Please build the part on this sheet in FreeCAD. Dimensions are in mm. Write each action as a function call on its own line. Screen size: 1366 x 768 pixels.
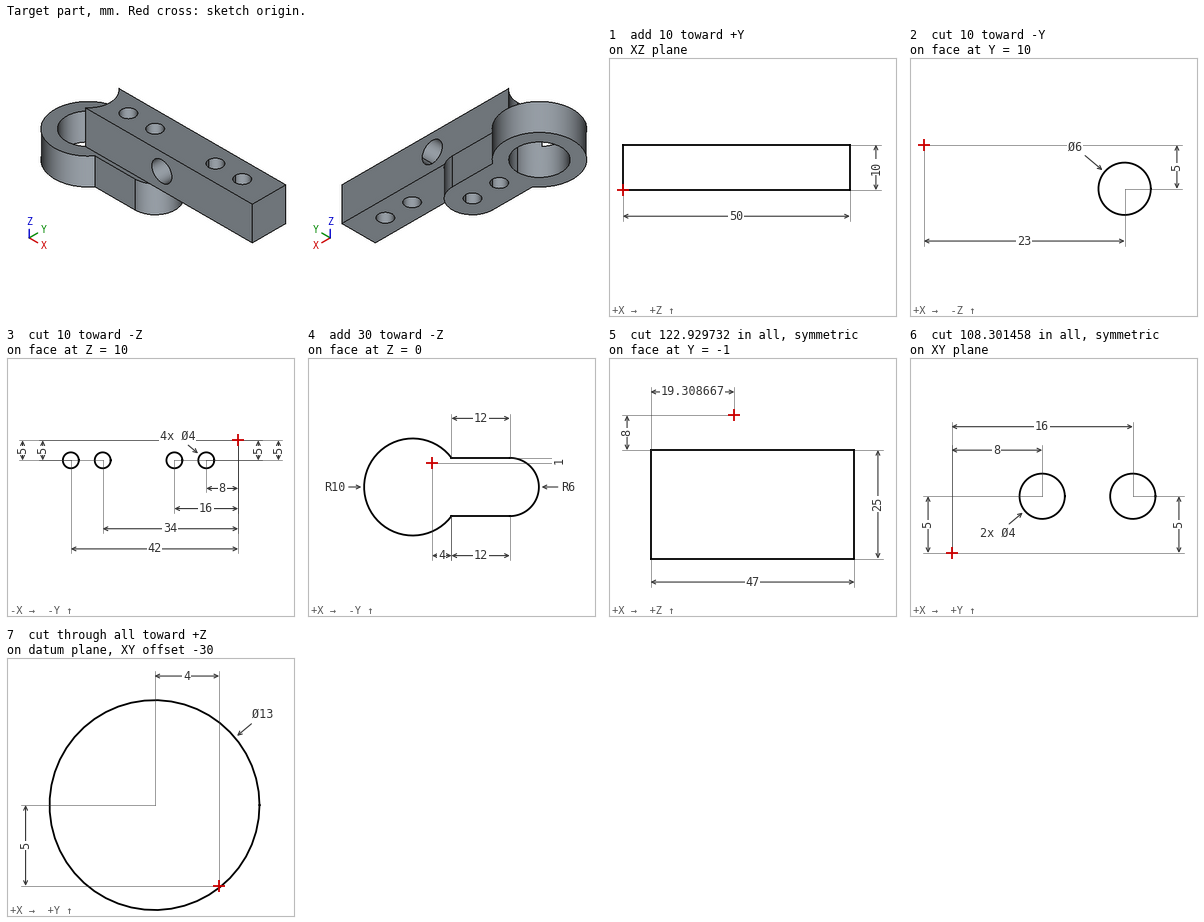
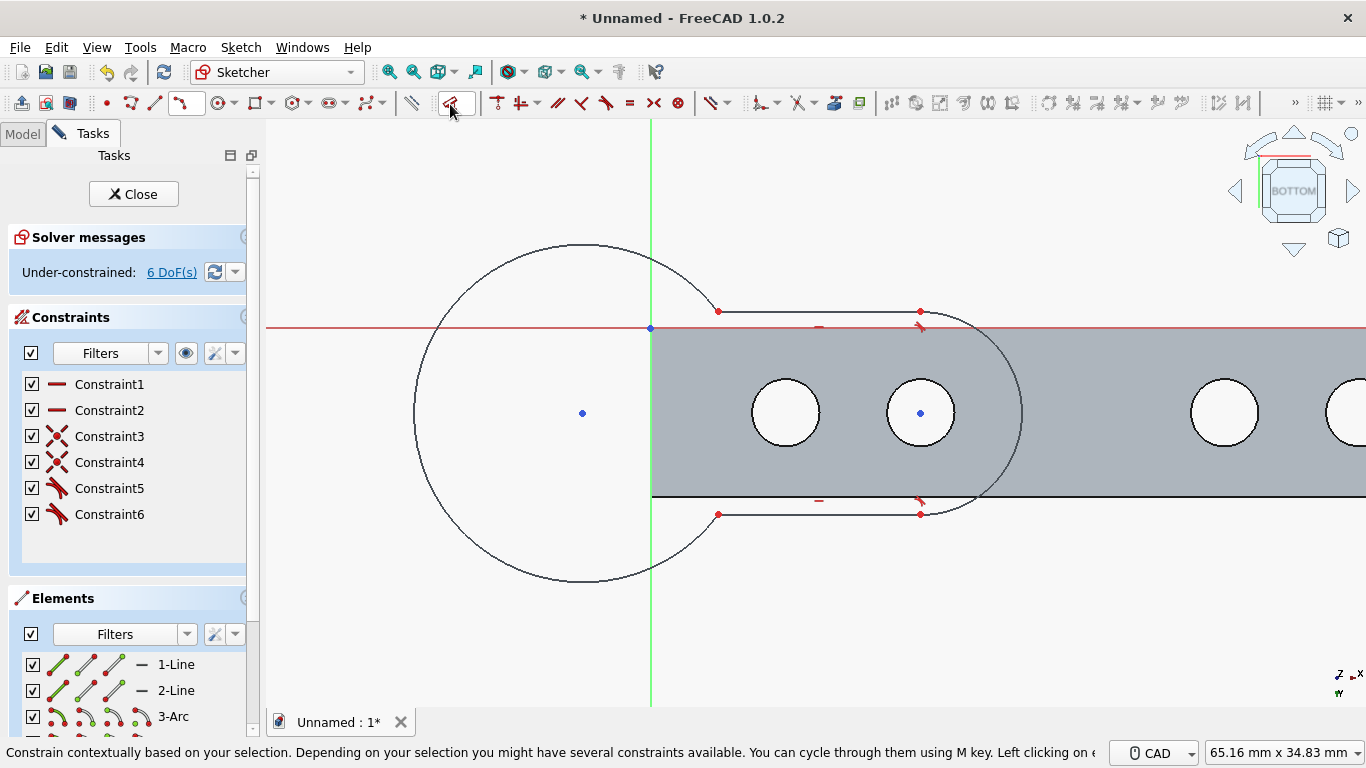
click(1003, 473)
click(1029, 492)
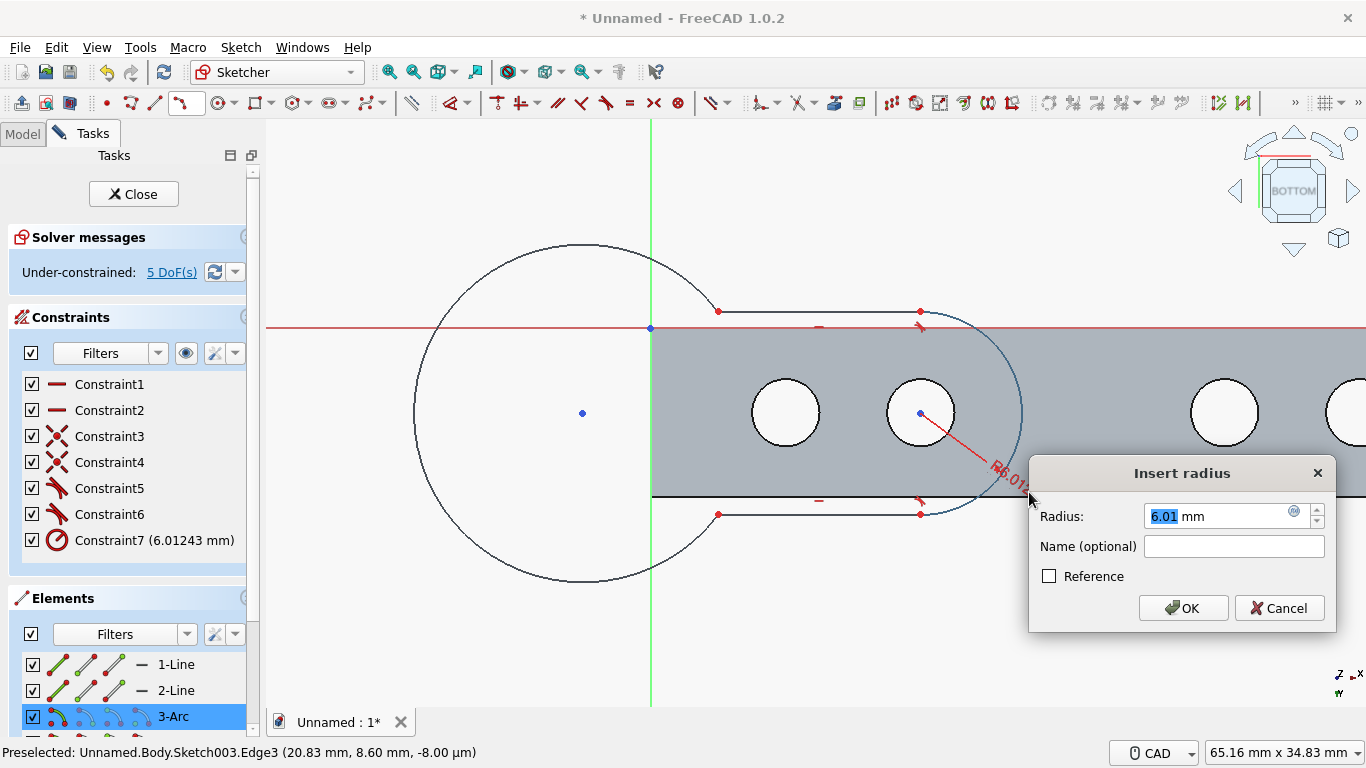
text(6)
key(Return)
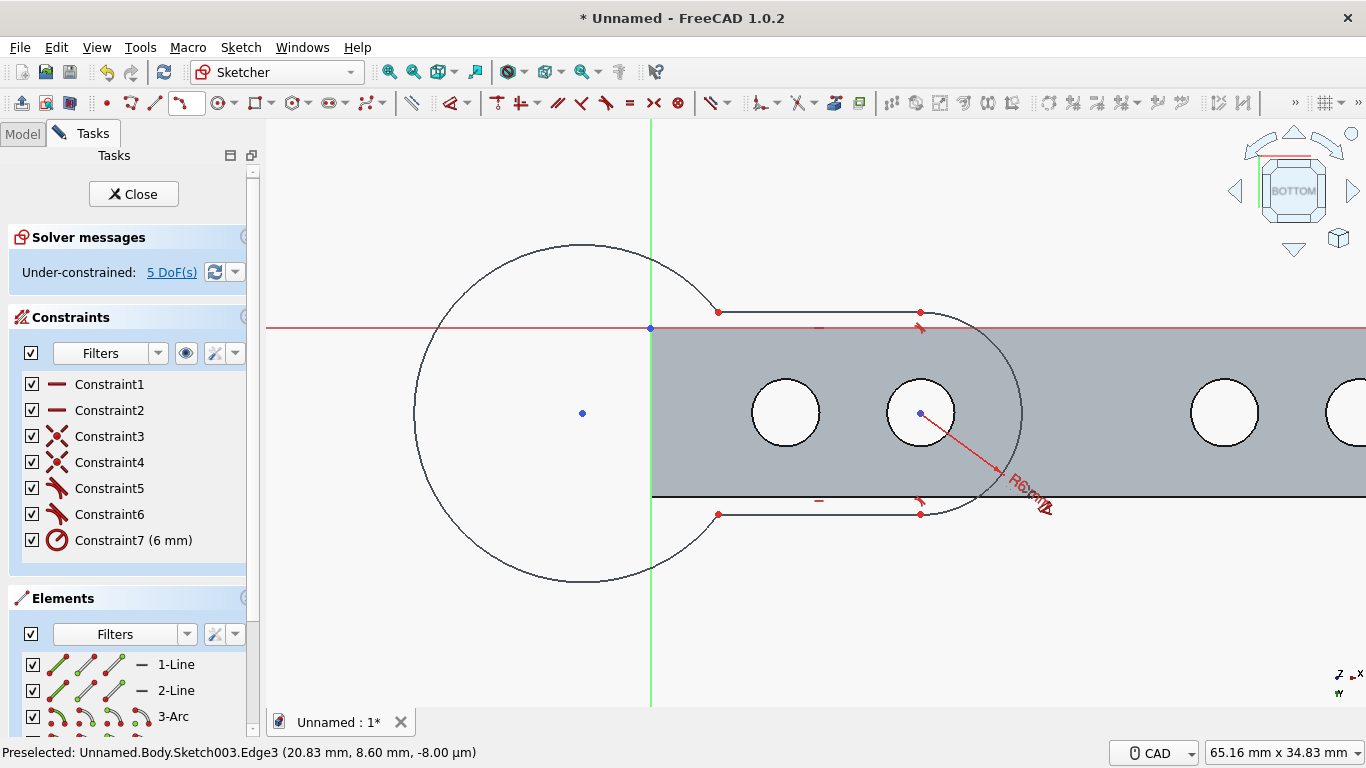
click(492, 272)
click(475, 245)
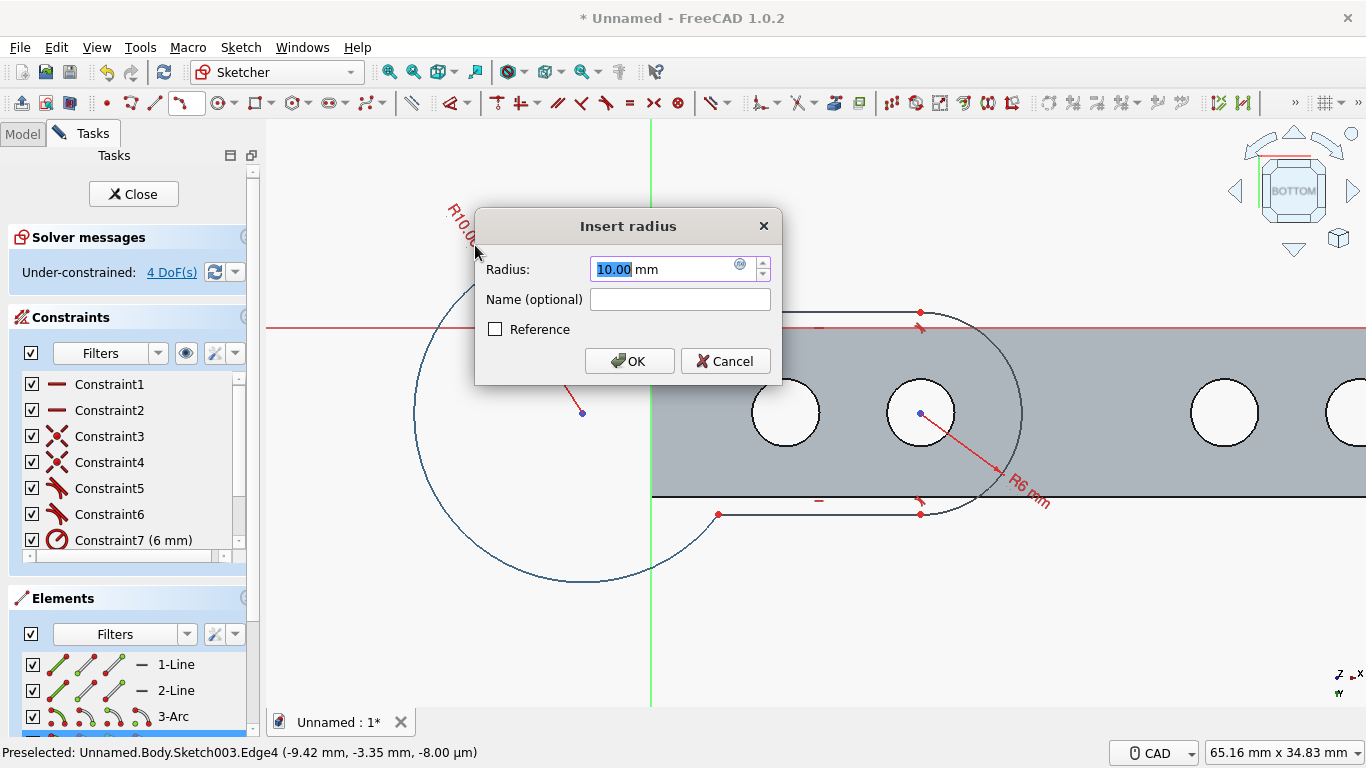
text(10)
key(Return)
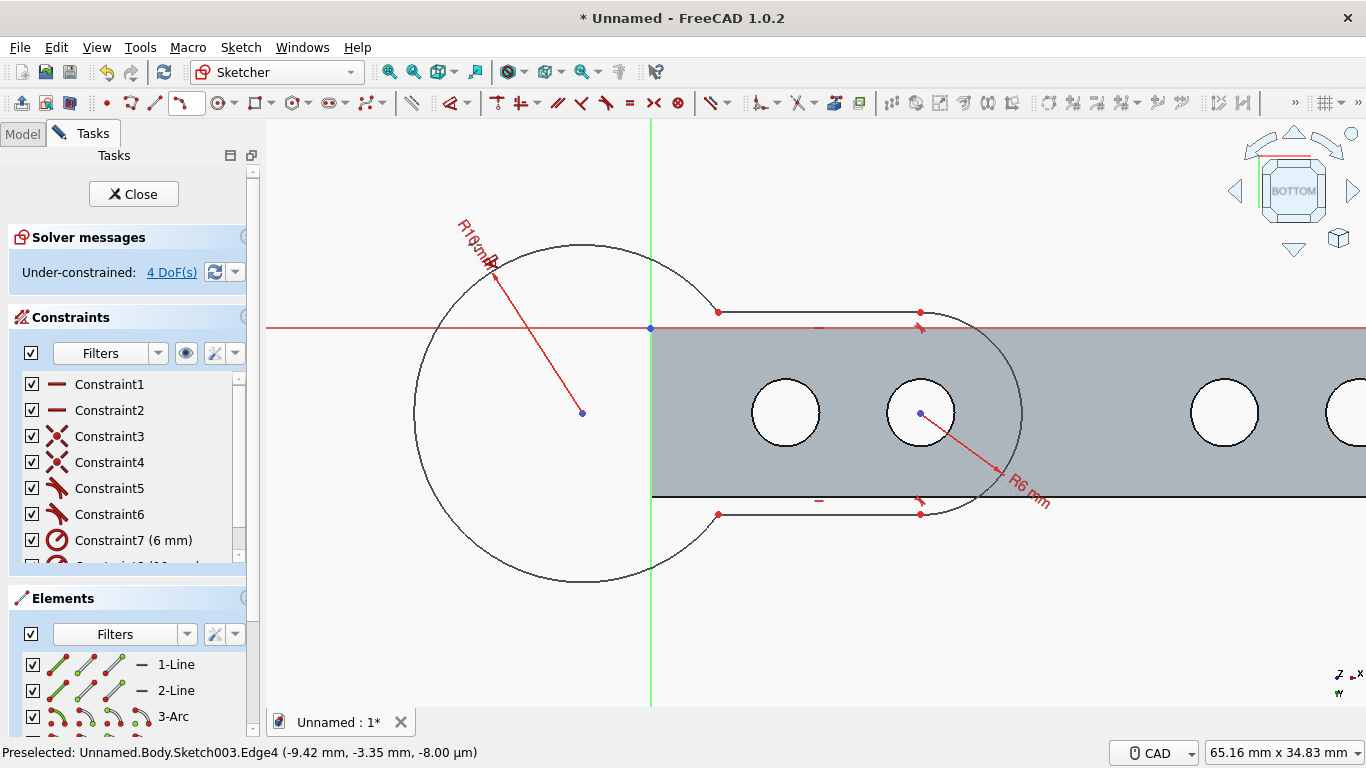
click(779, 515)
click(819, 549)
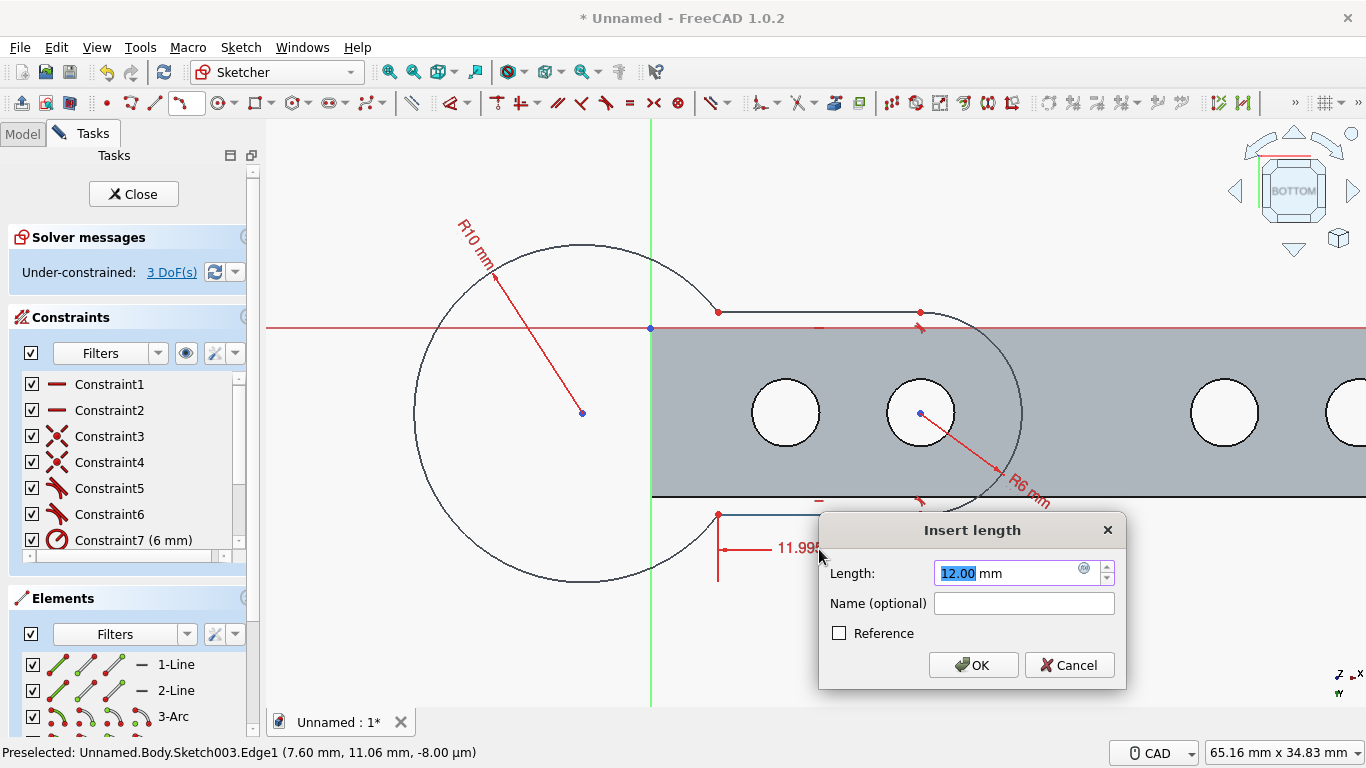
text(12)
key(Return)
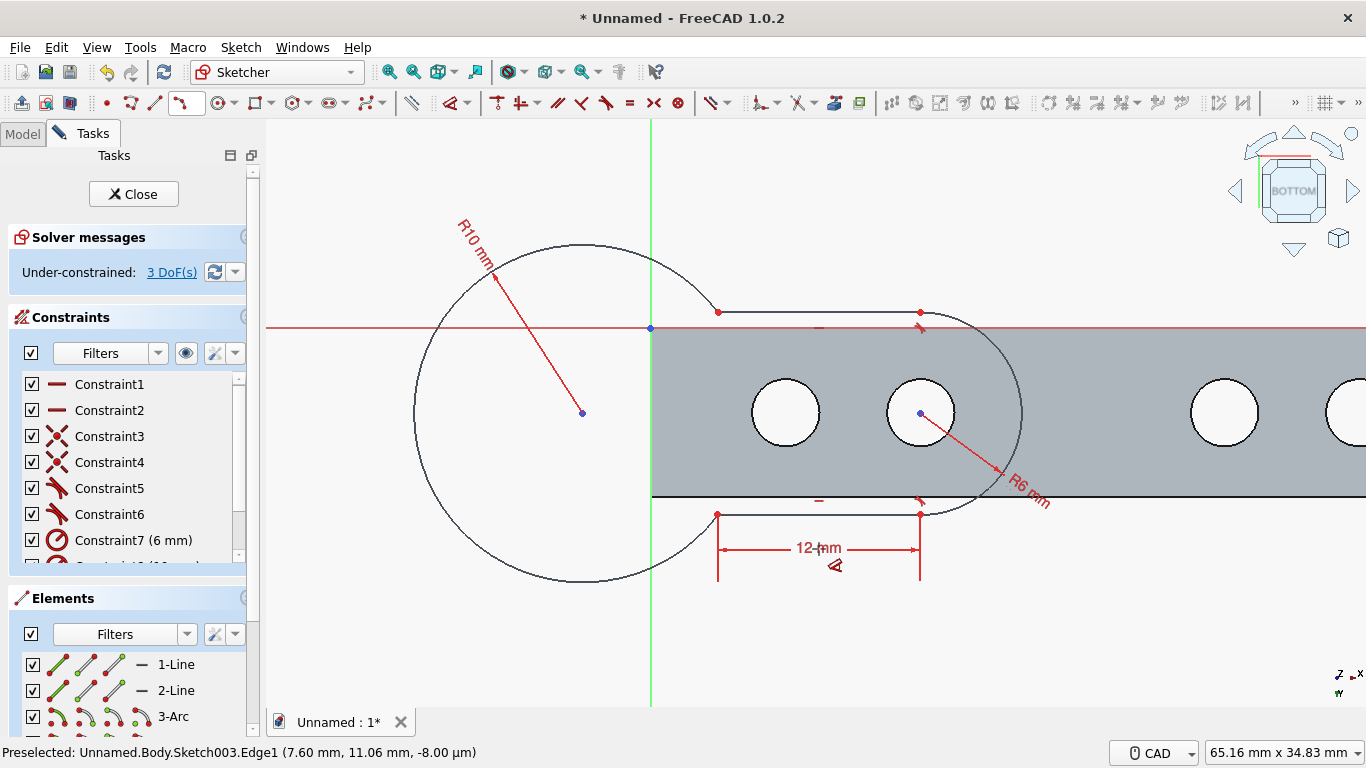
click(860, 312)
click(819, 278)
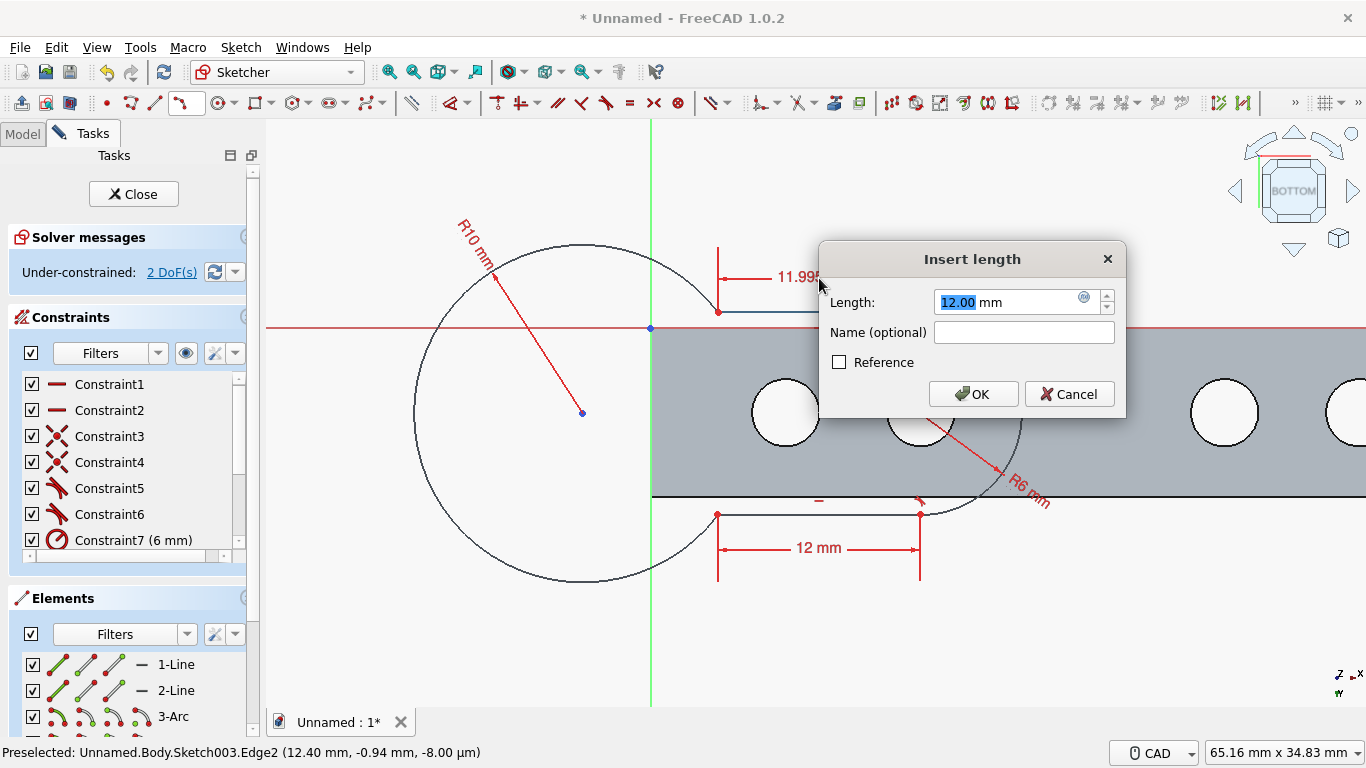
text(12)
key(Return)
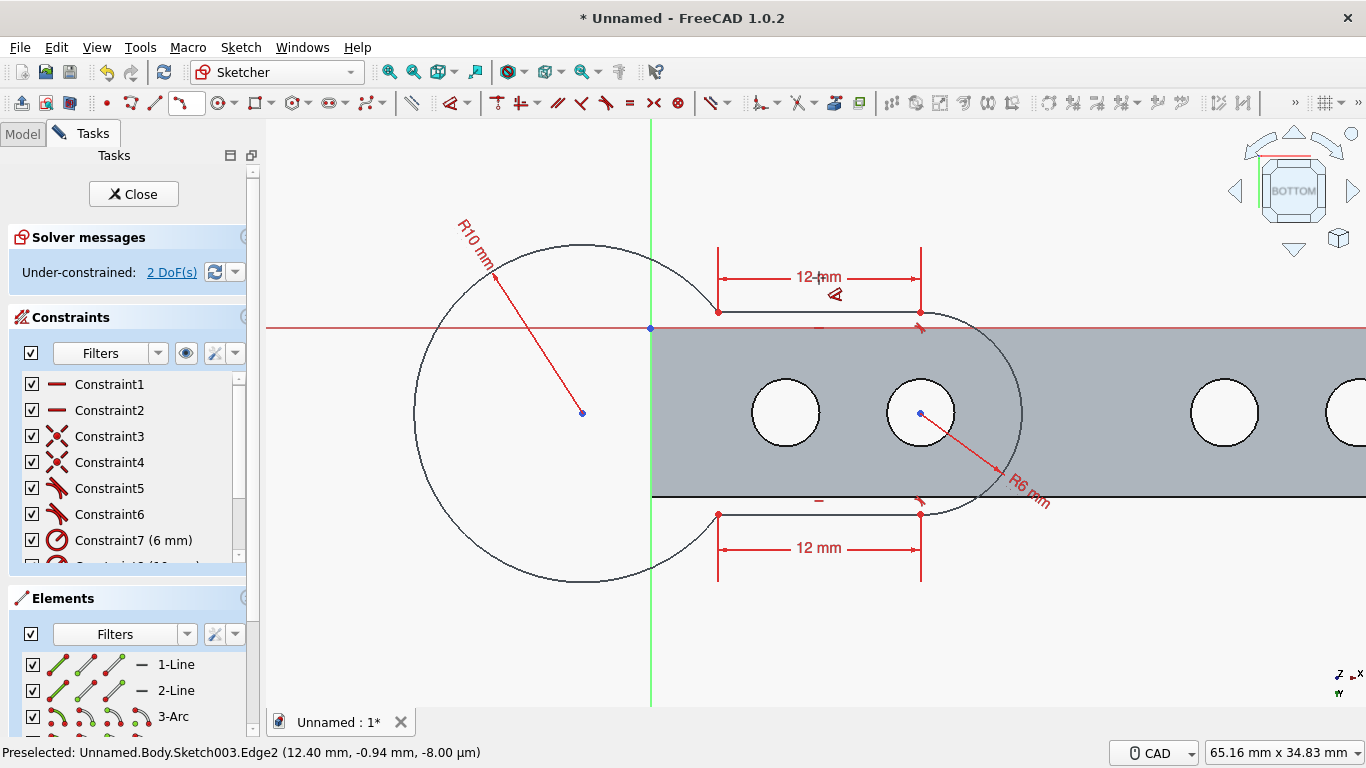
click(718, 515)
click(708, 549)